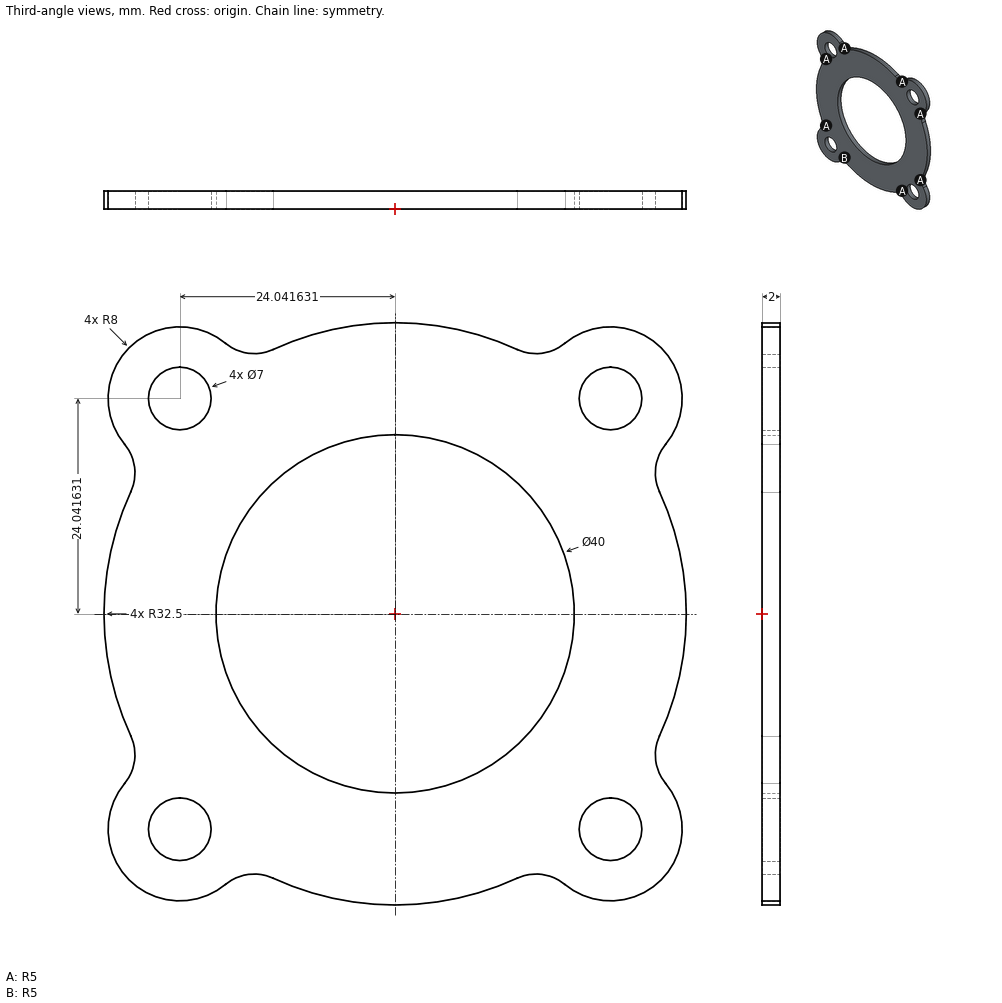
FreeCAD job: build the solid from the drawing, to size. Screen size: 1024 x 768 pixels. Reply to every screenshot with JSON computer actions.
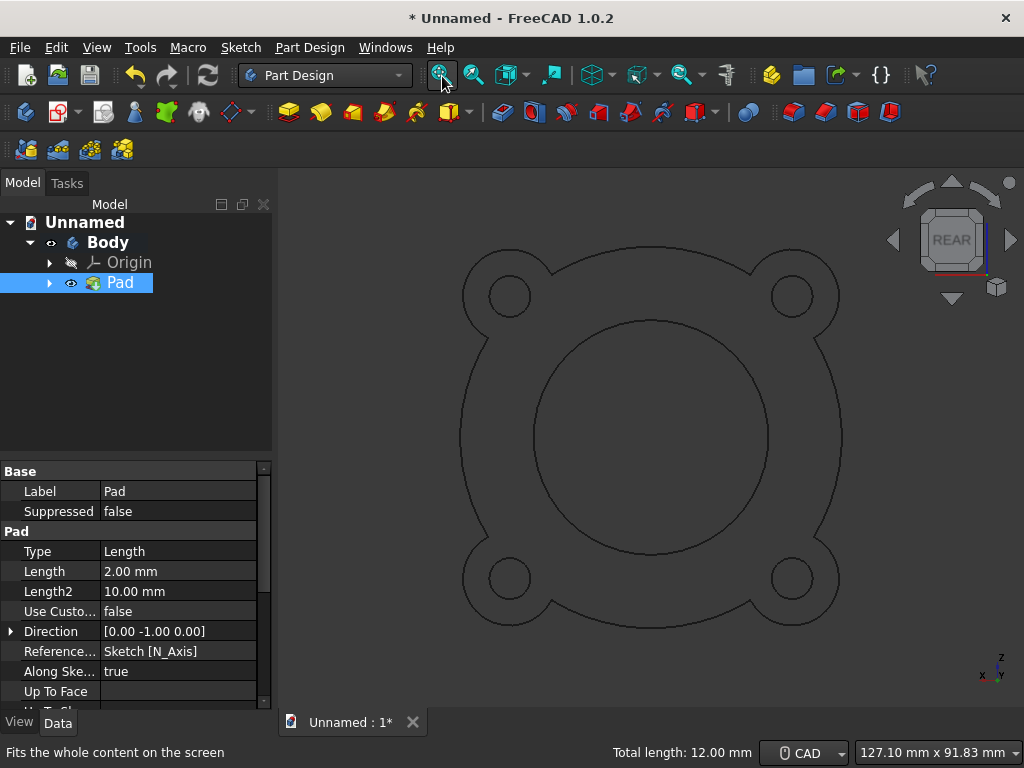
{"action": "key", "text": "6"}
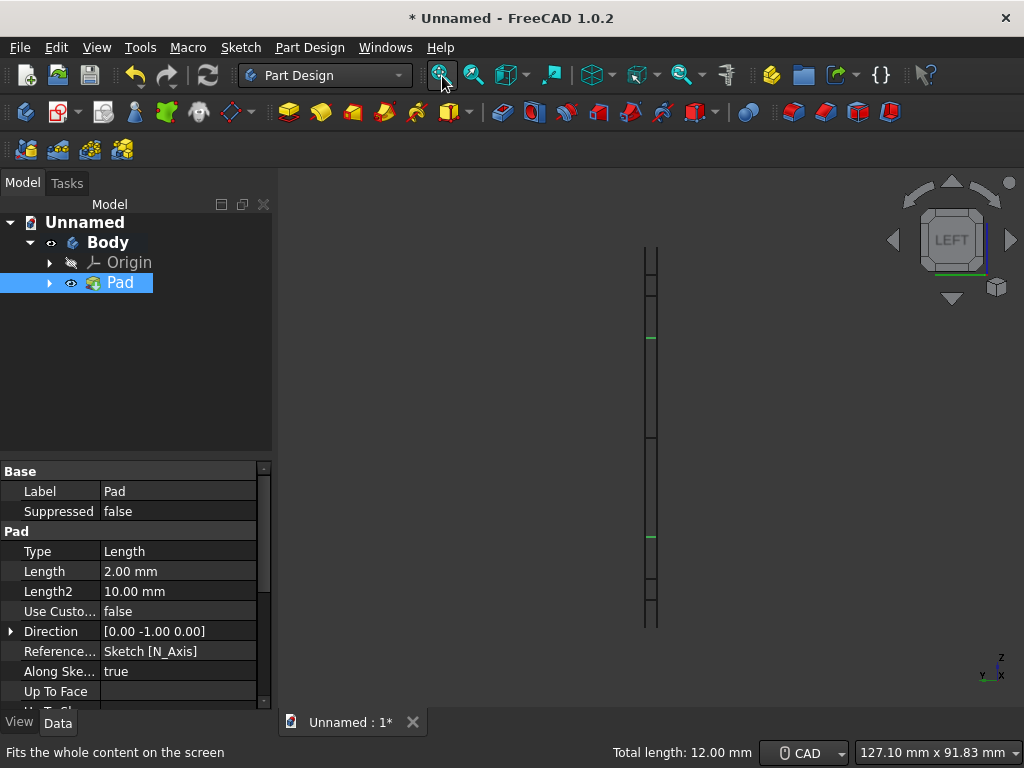
{"action": "scroll", "coordinate": [651, 274], "scroll_direction": "up", "scroll_amount": 7}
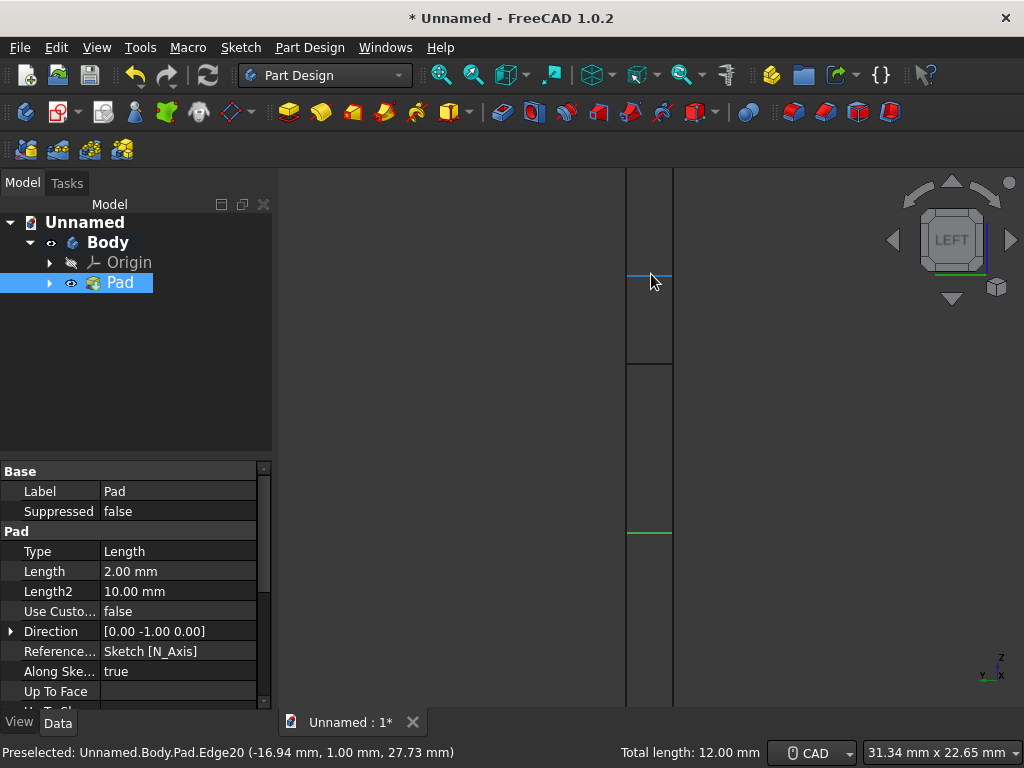
{"action": "left_click", "coordinate": [649, 275], "text": "ctrl"}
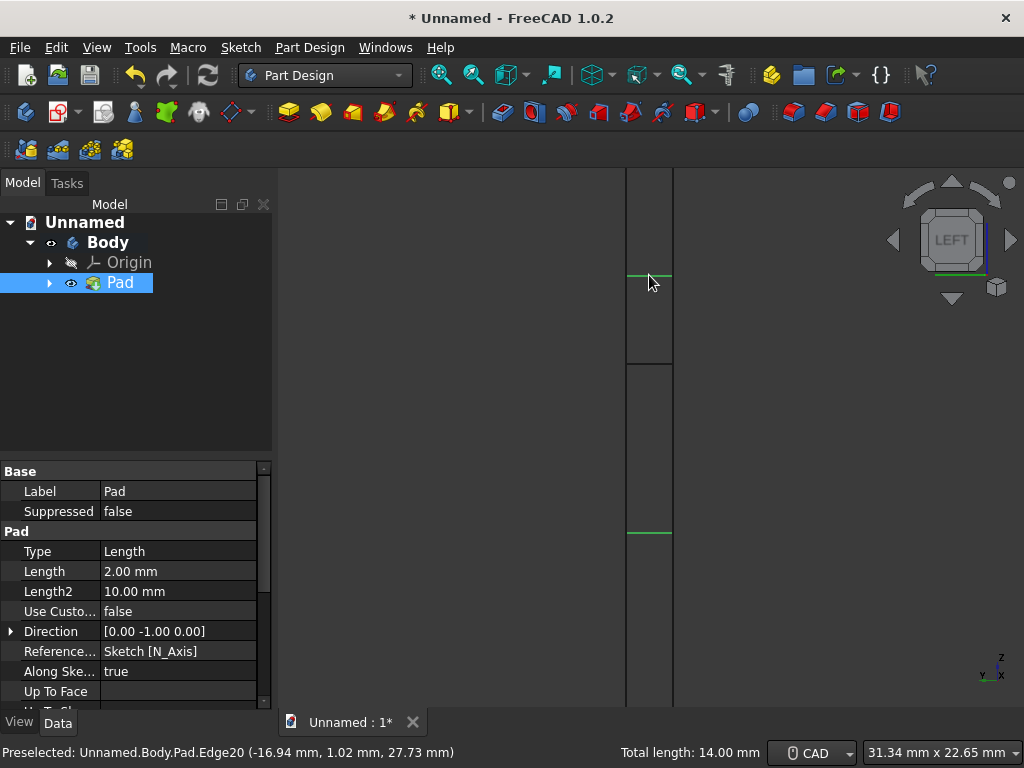
{"action": "key", "text": "v 1"}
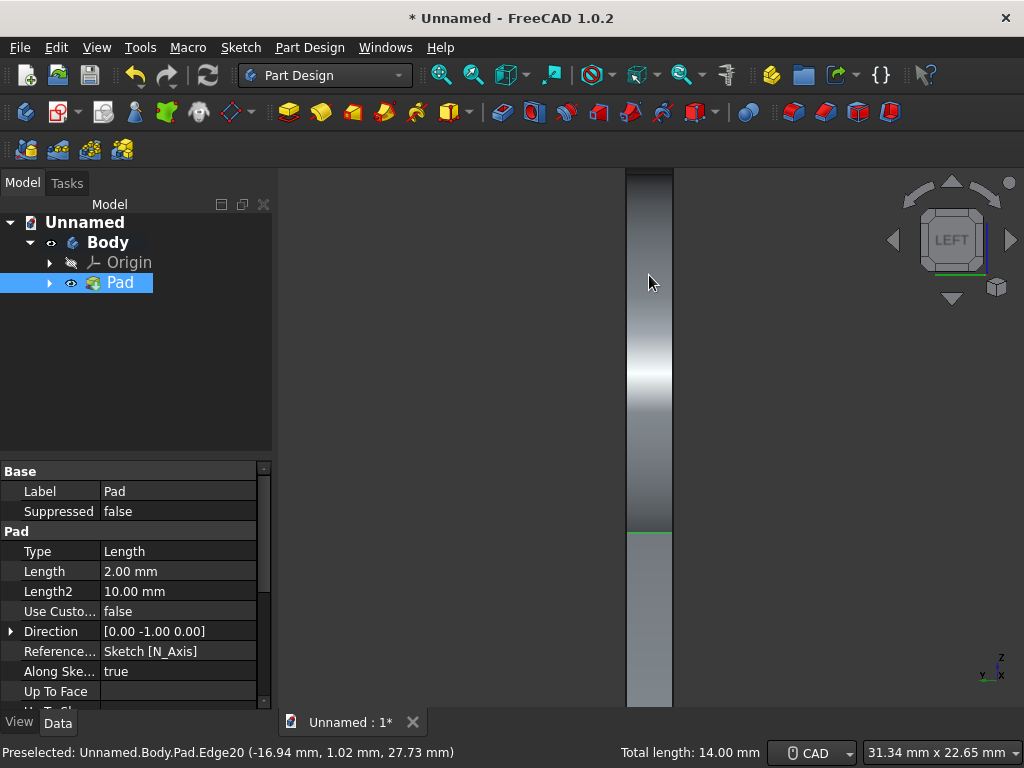
{"action": "left_click", "coordinate": [794, 112]}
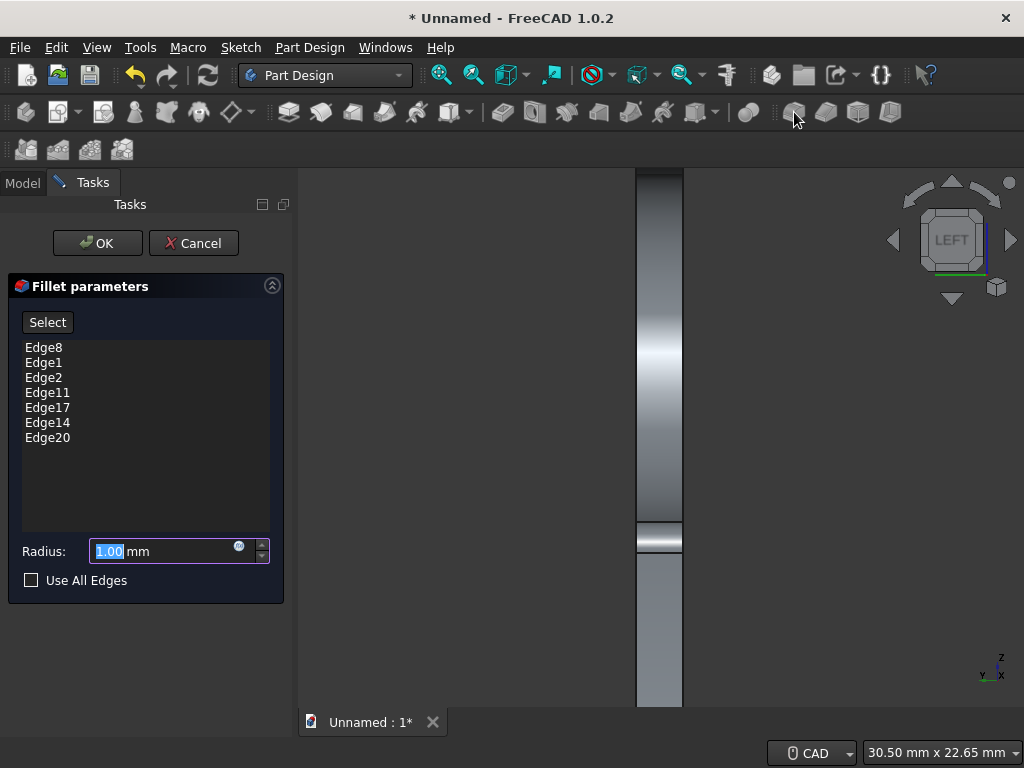
{"action": "type", "text": "5"}
{"action": "key", "text": "Tab"}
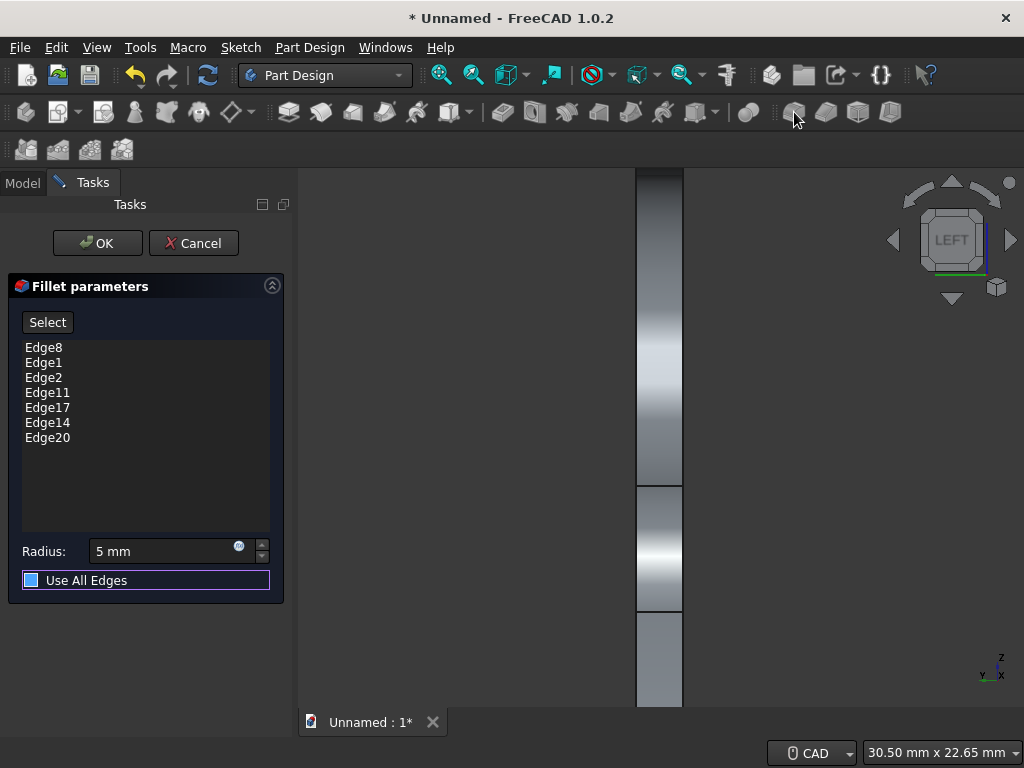
{"action": "left_click", "coordinate": [98, 243]}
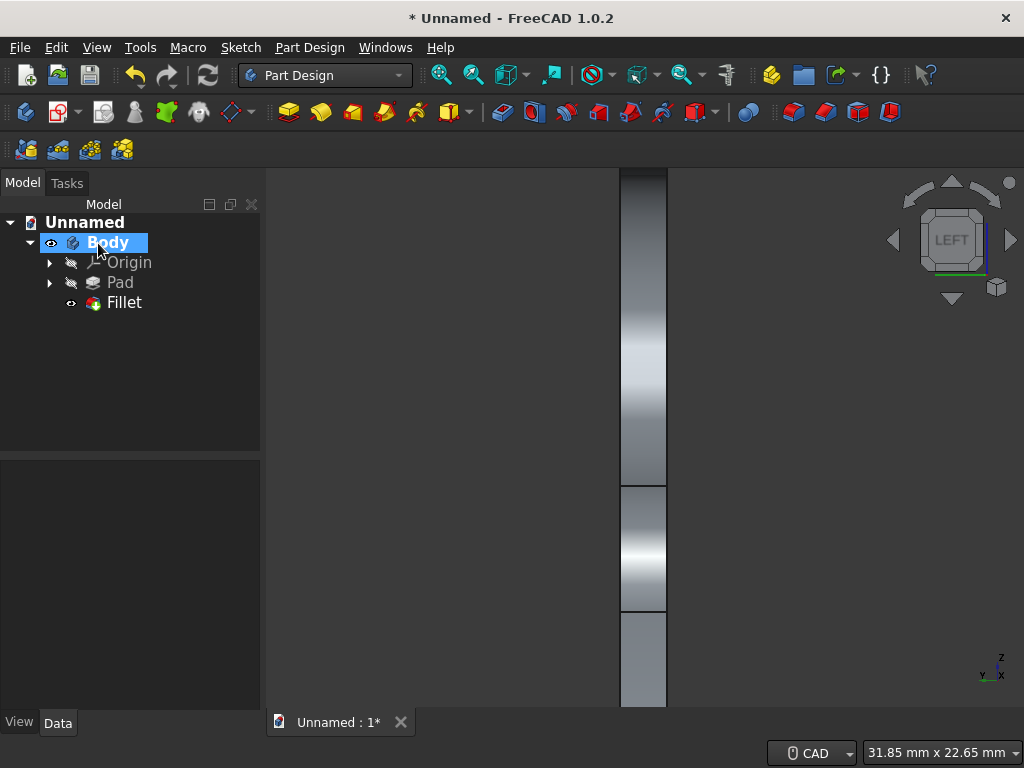
{"action": "key", "text": "v f"}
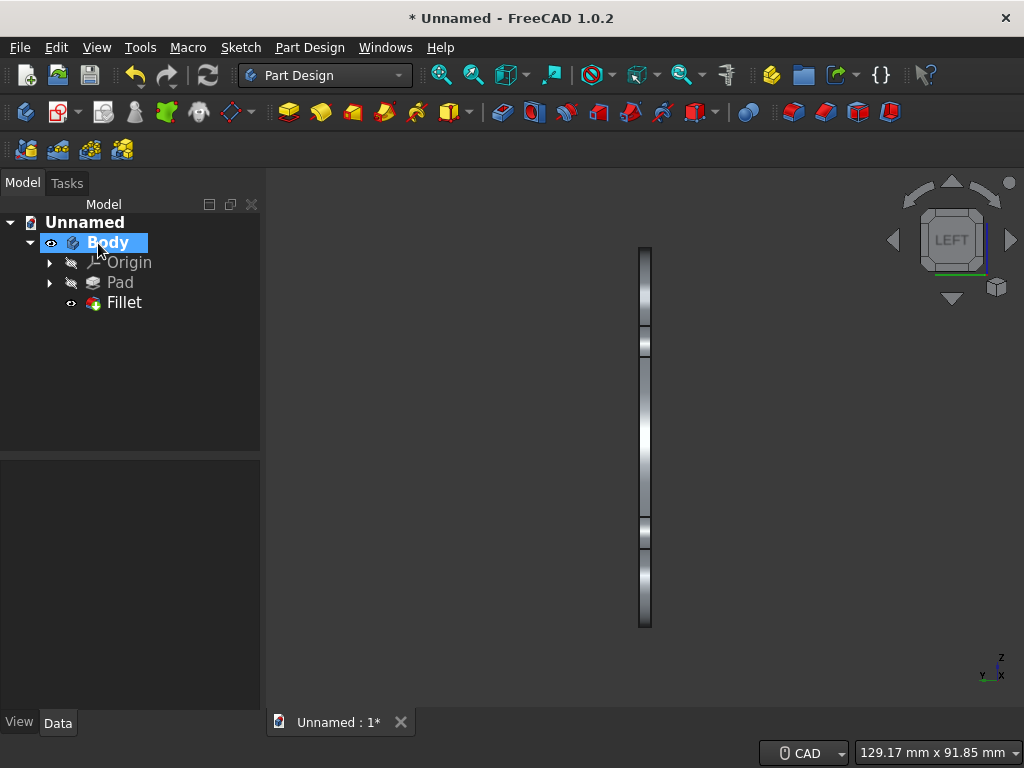
{"action": "scroll", "coordinate": [645, 599], "scroll_direction": "up", "scroll_amount": 7}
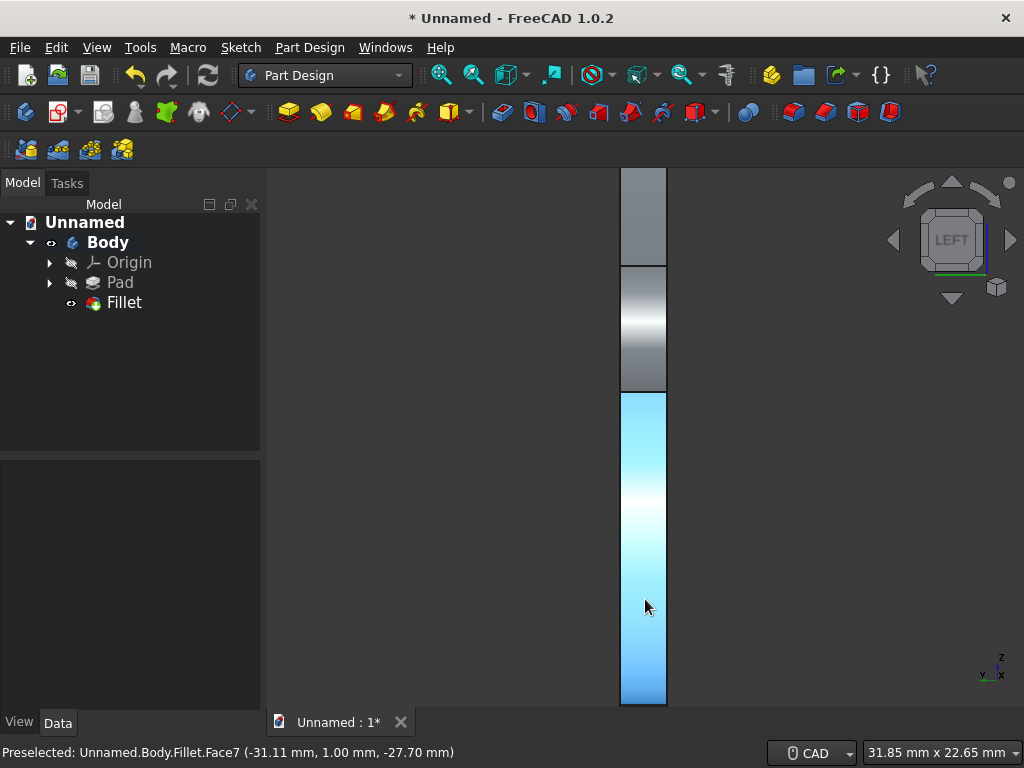
{"action": "key", "text": "v f"}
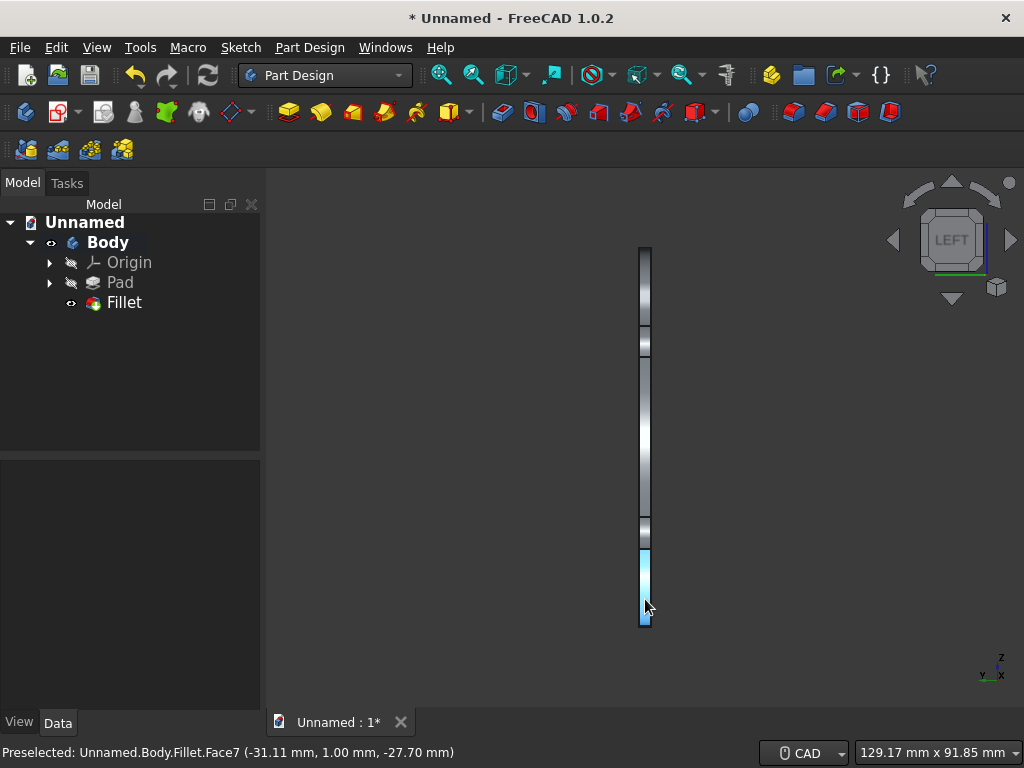
{"action": "key", "text": "0"}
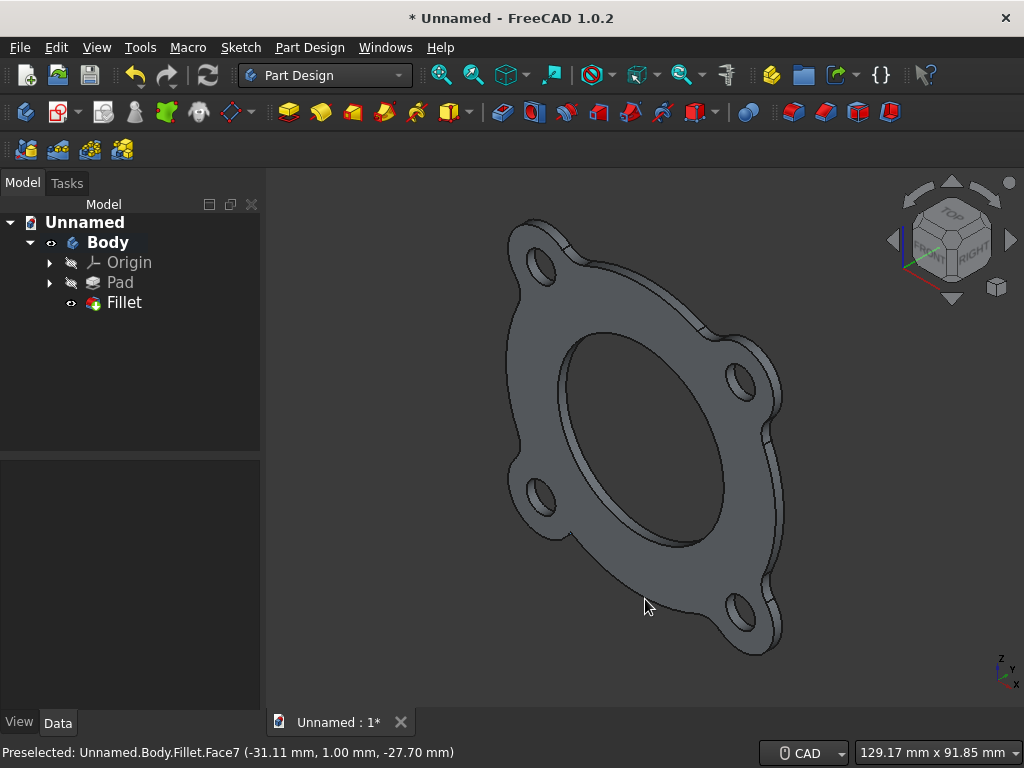
{"action": "scroll", "coordinate": [575, 529], "scroll_direction": "up", "scroll_amount": 7}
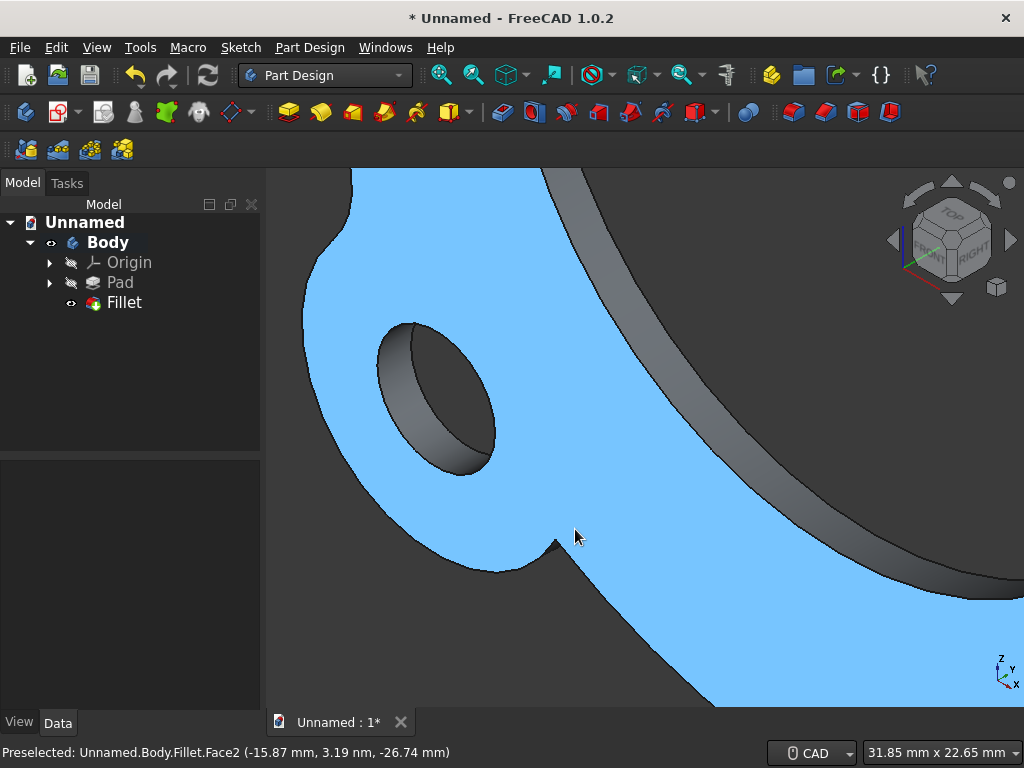
{"action": "left_click", "coordinate": [442, 76]}